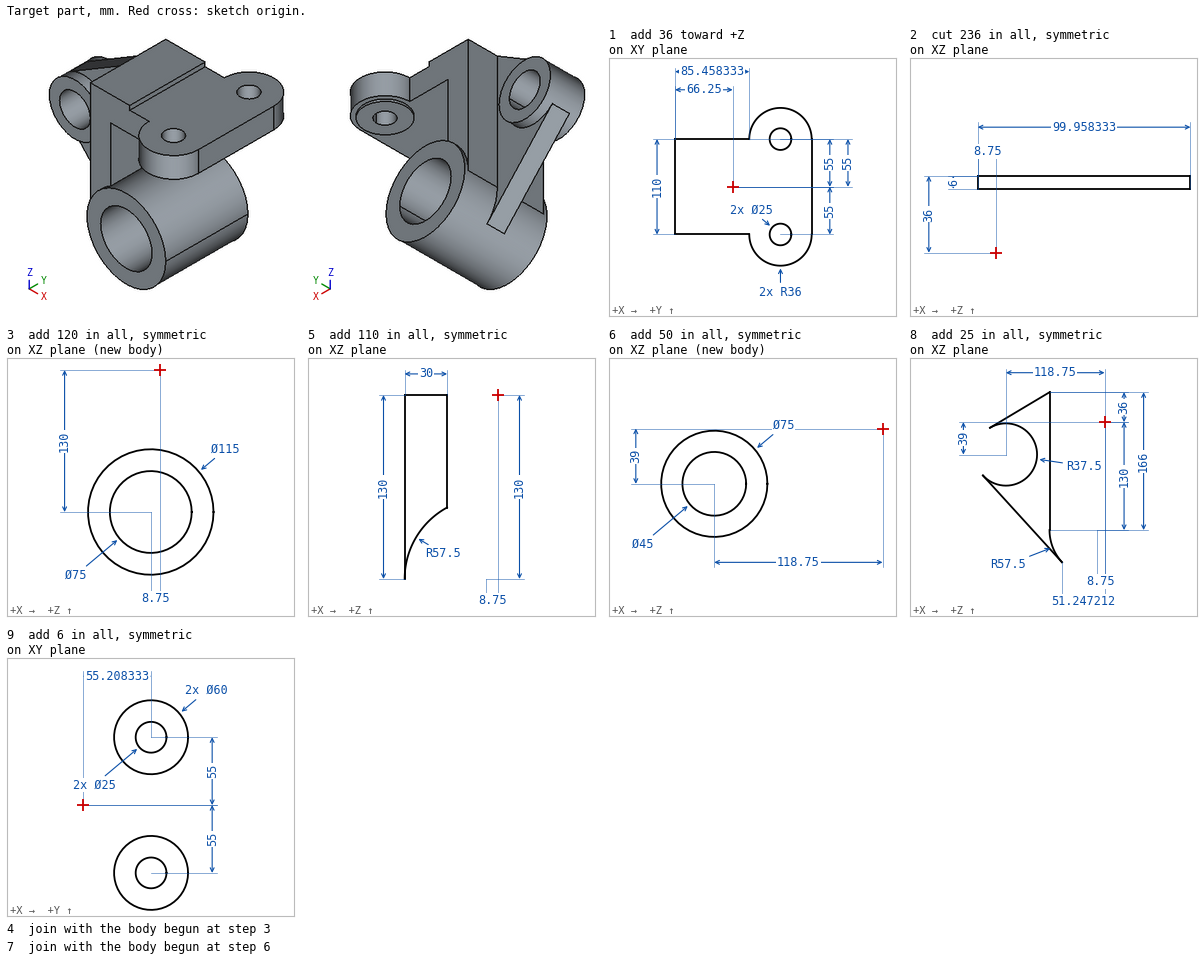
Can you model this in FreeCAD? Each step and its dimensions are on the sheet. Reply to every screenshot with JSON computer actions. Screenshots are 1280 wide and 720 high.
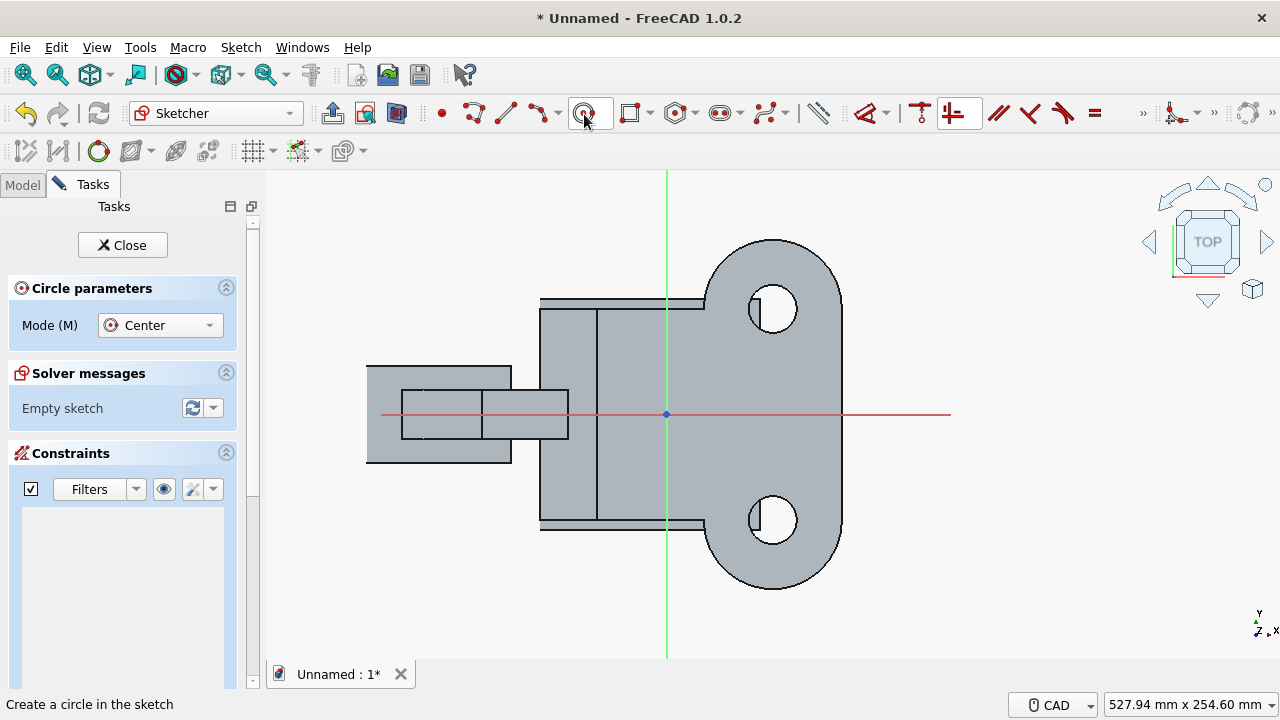
{"action": "left_click", "coordinate": [773, 309]}
{"action": "left_click", "coordinate": [814, 268]}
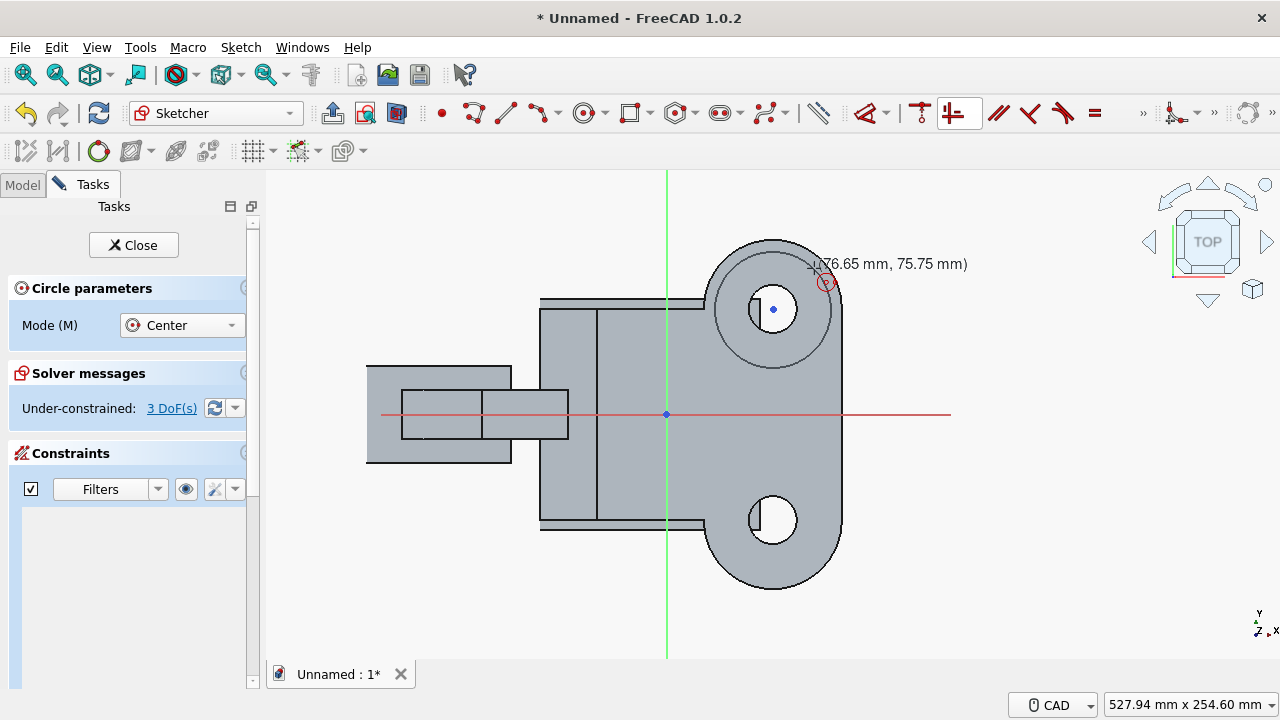
{"action": "left_click", "coordinate": [773, 520]}
{"action": "left_click", "coordinate": [814, 479]}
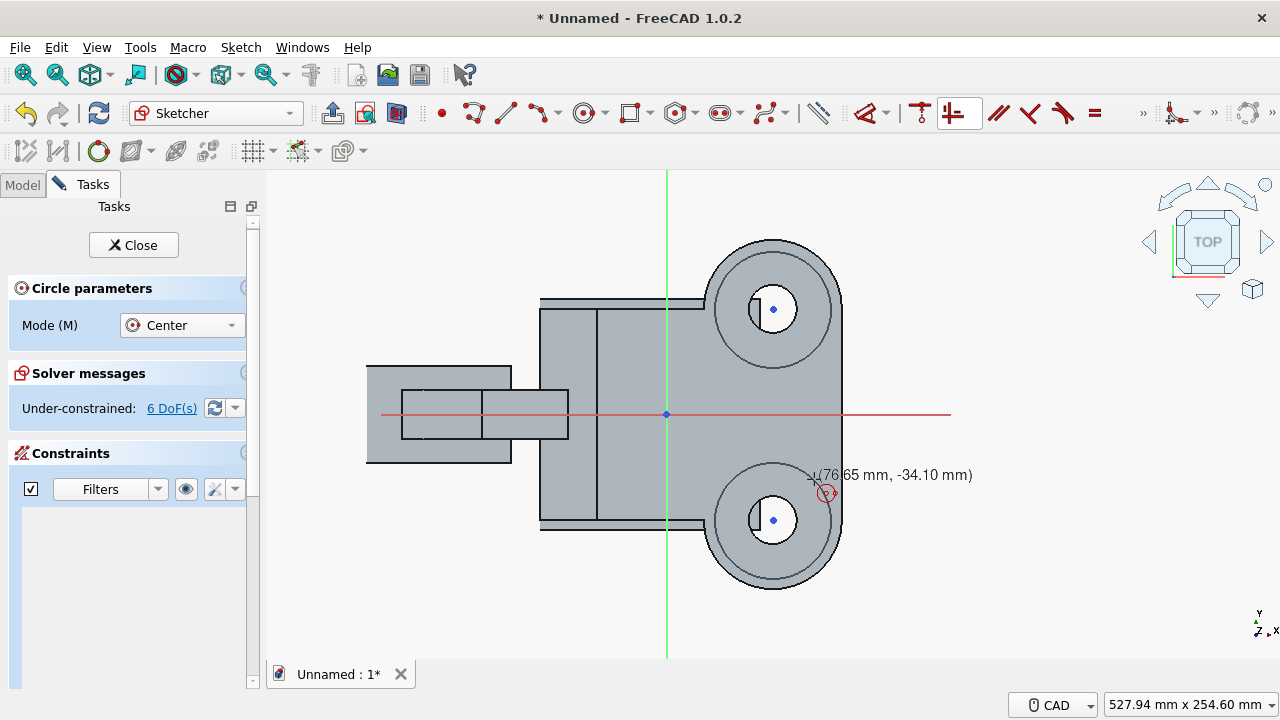
{"action": "left_click", "coordinate": [773, 310]}
{"action": "left_click", "coordinate": [790, 292]}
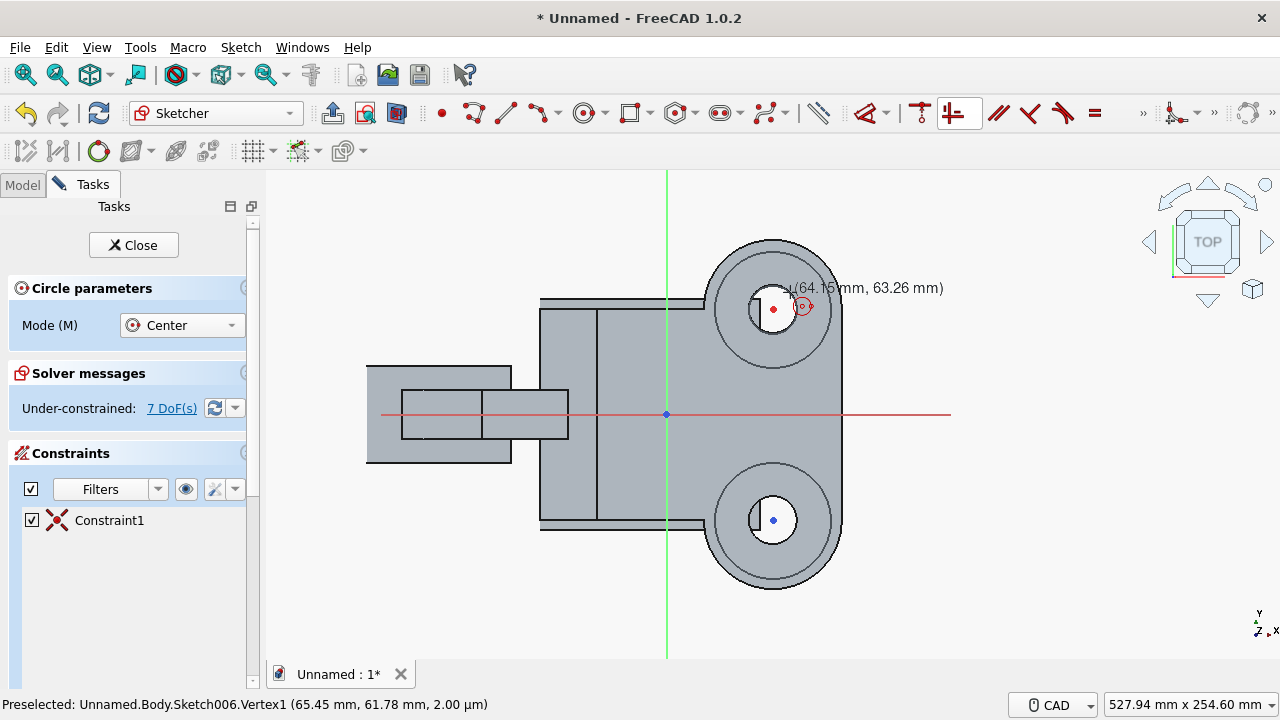
{"action": "left_click", "coordinate": [773, 521]}
{"action": "left_click", "coordinate": [790, 503]}
{"action": "key", "text": "Escape"}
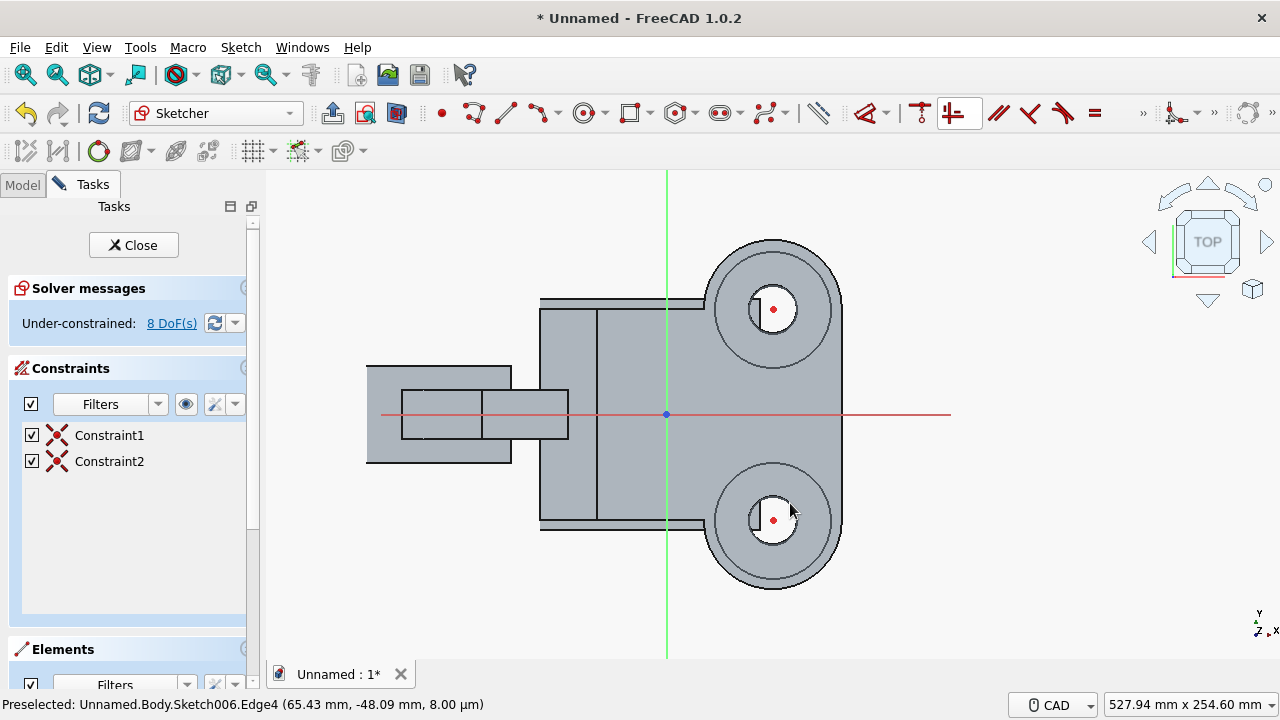
{"action": "left_click", "coordinate": [814, 269]}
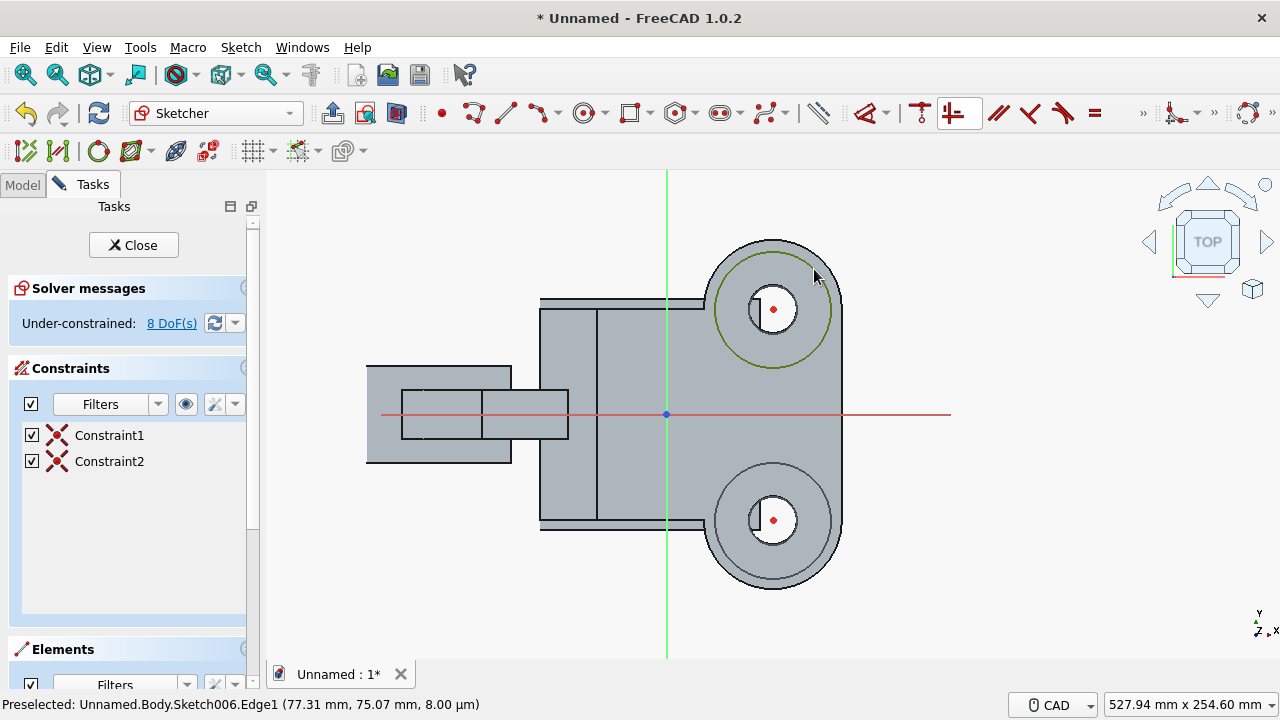
{"action": "left_click", "coordinate": [814, 480]}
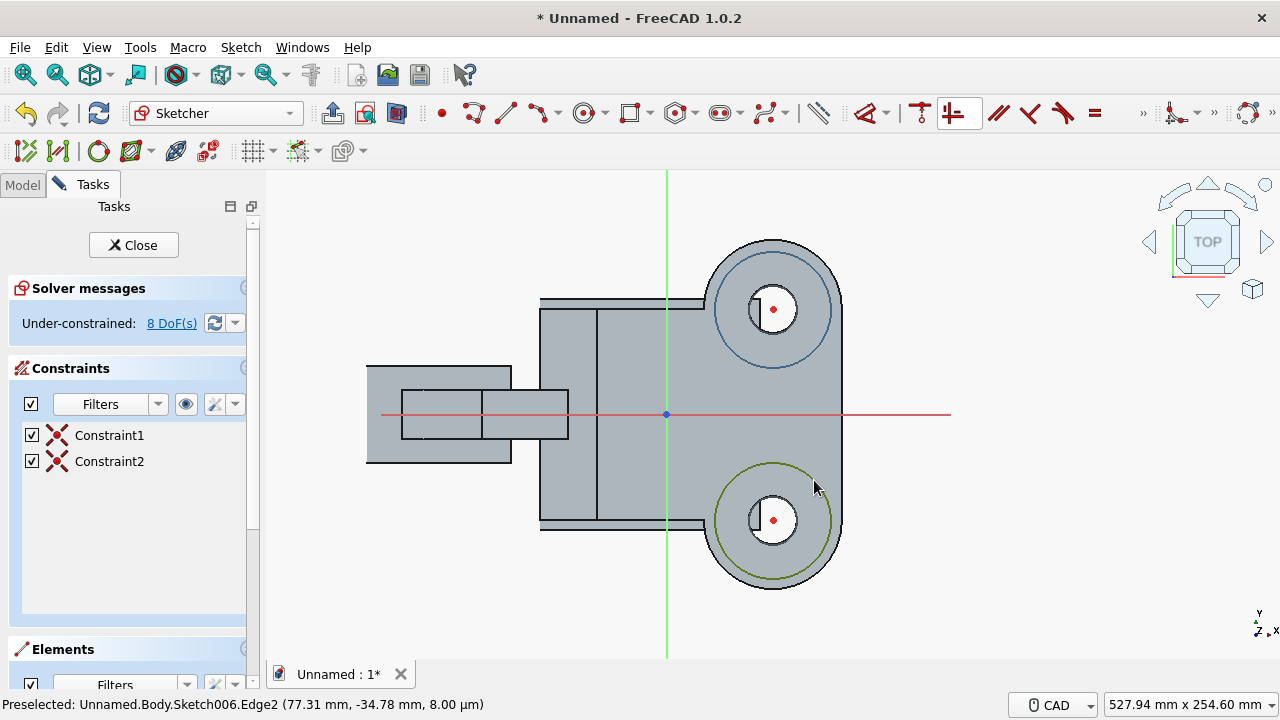
{"action": "left_click", "coordinate": [1096, 114]}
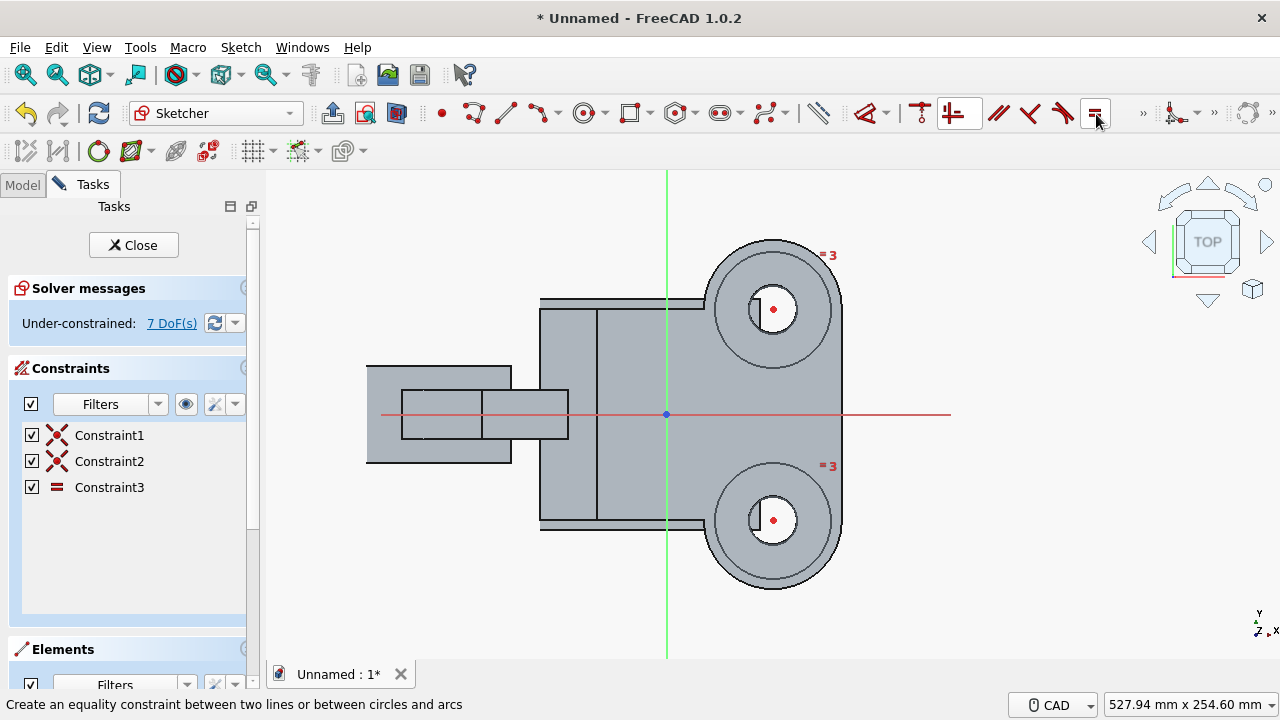
{"action": "left_click", "coordinate": [790, 293]}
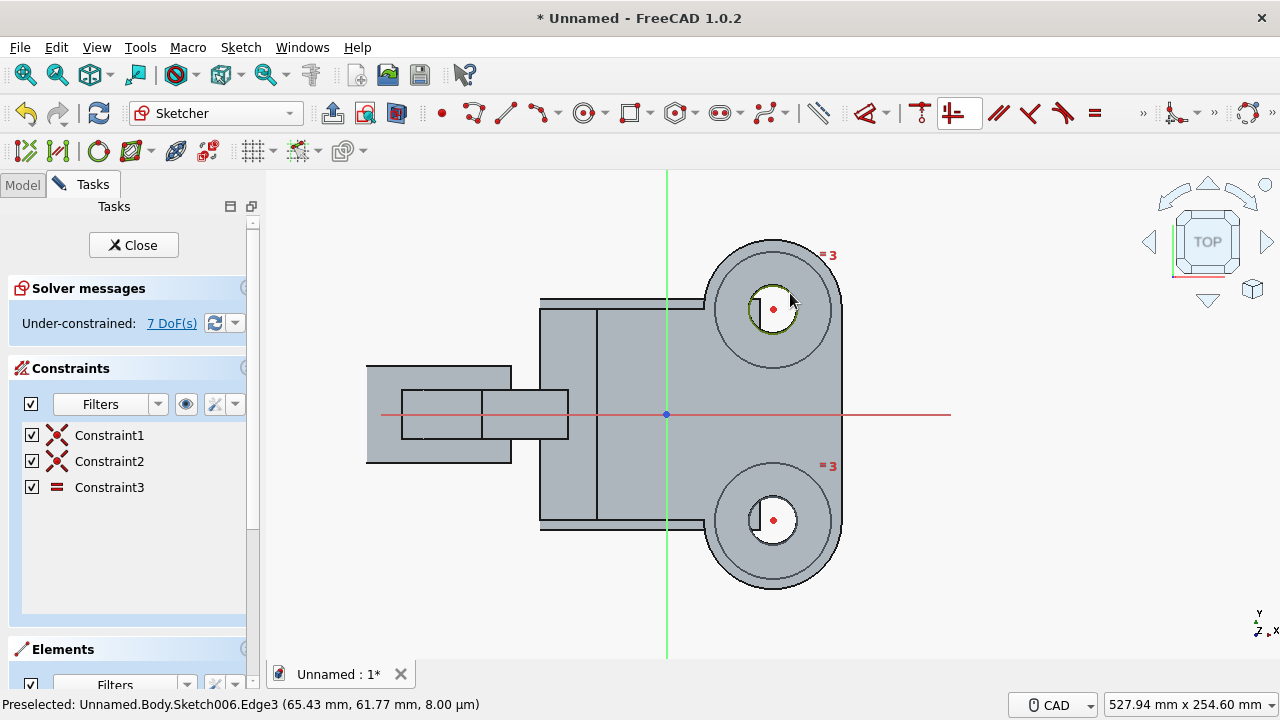
{"action": "left_click", "coordinate": [790, 504]}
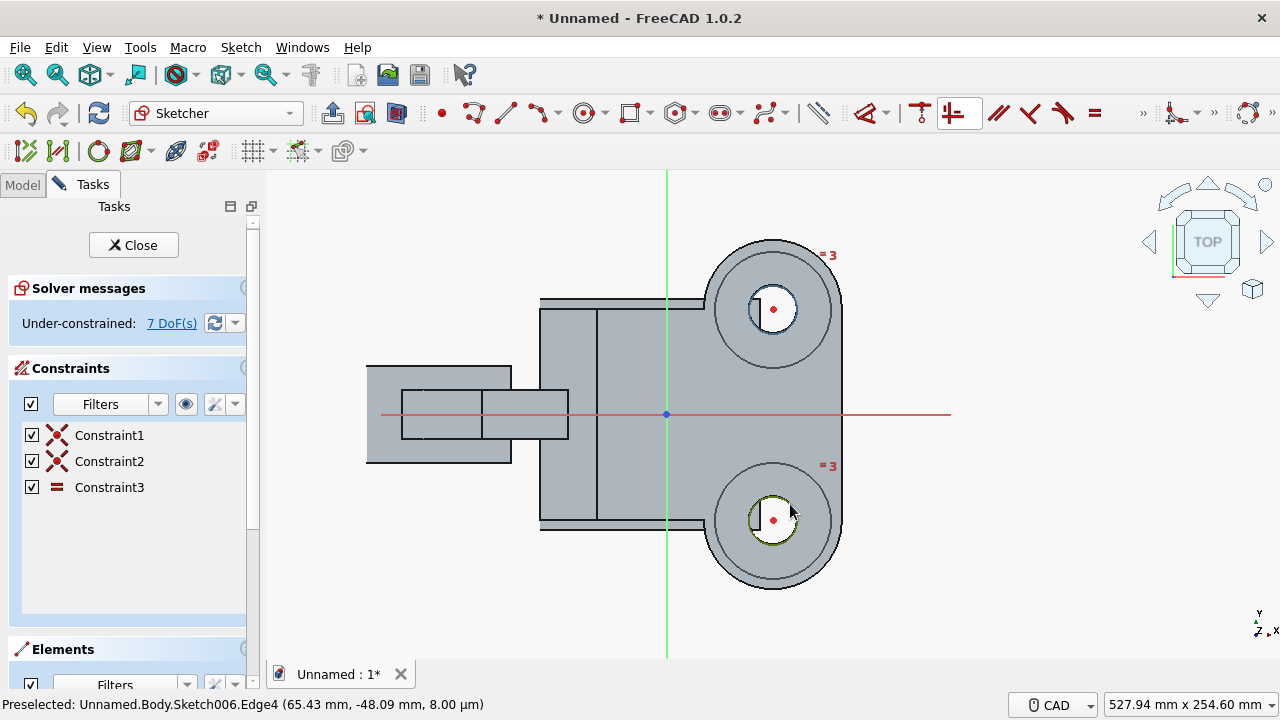
{"action": "left_click", "coordinate": [1096, 114]}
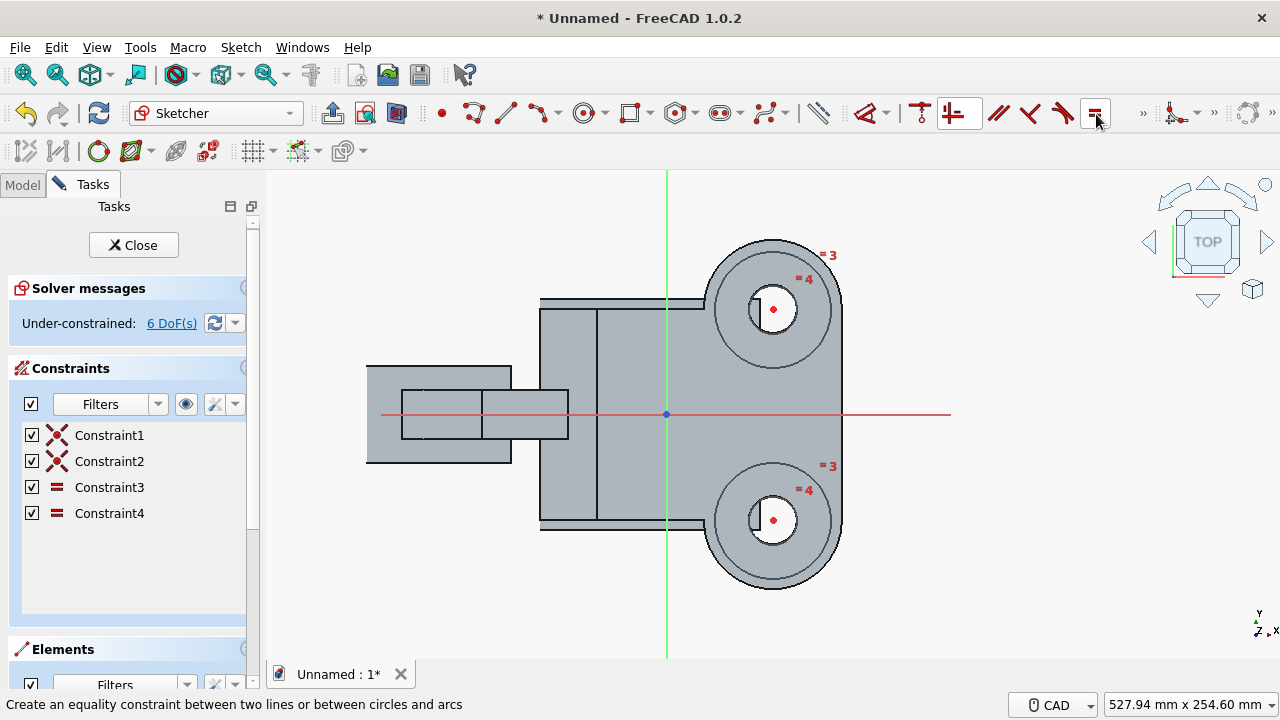
{"action": "left_click", "coordinate": [773, 310]}